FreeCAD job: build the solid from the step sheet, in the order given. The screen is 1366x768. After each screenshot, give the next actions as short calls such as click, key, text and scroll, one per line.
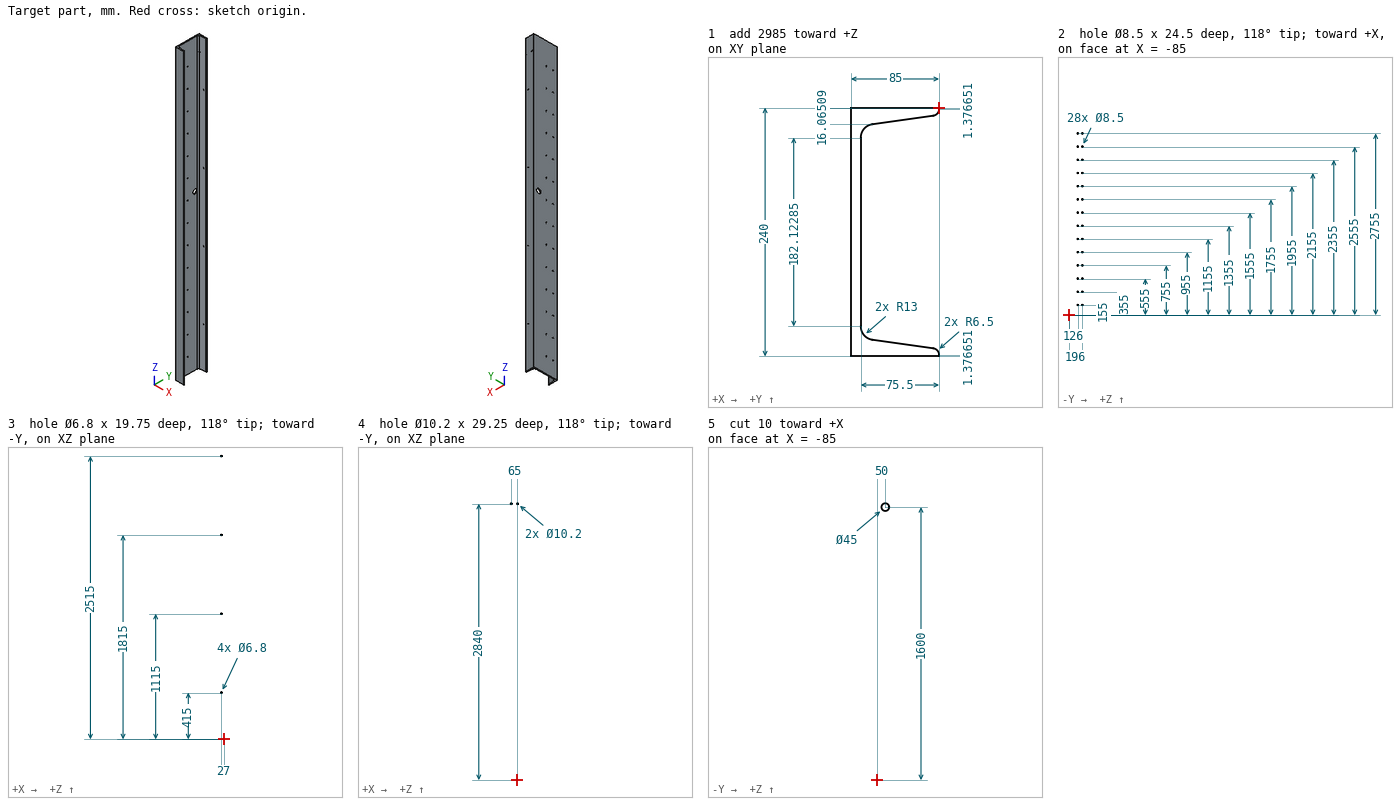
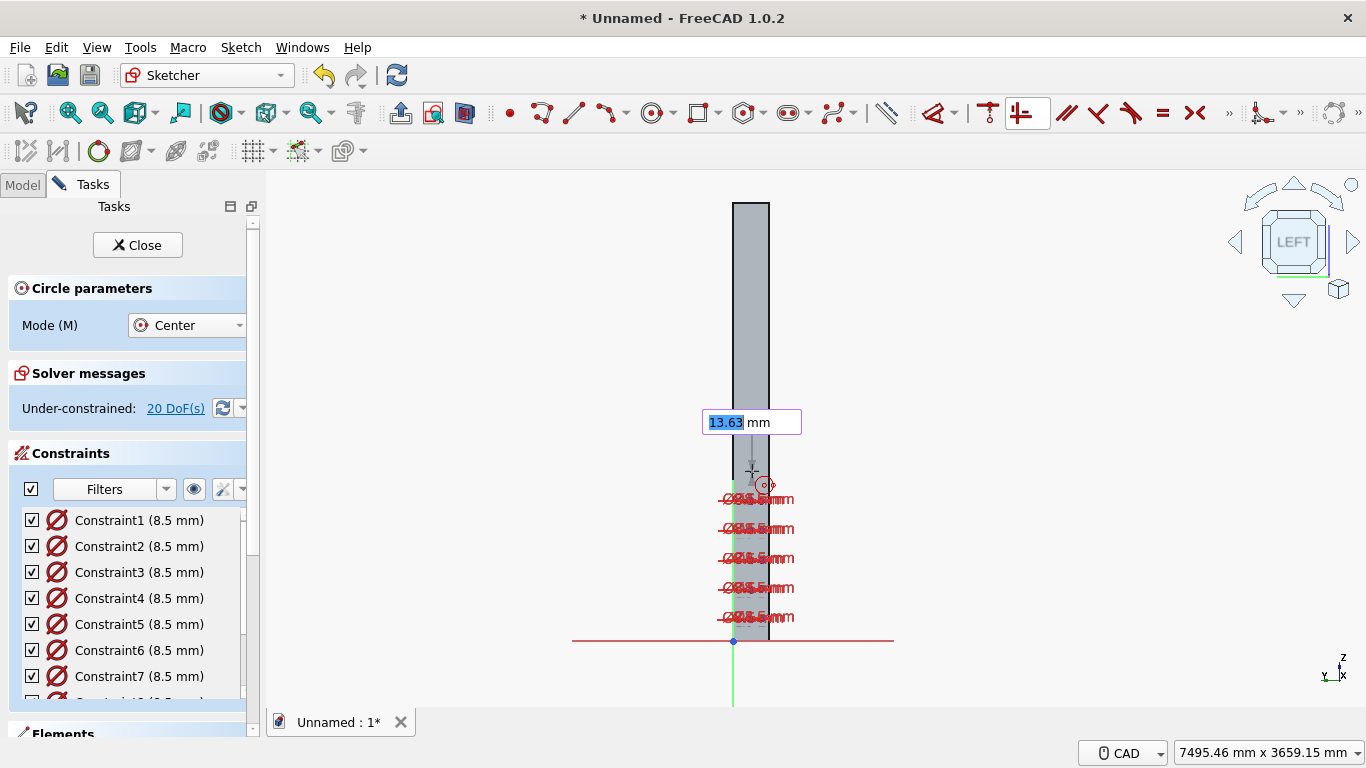
text(8.5)
key(Return)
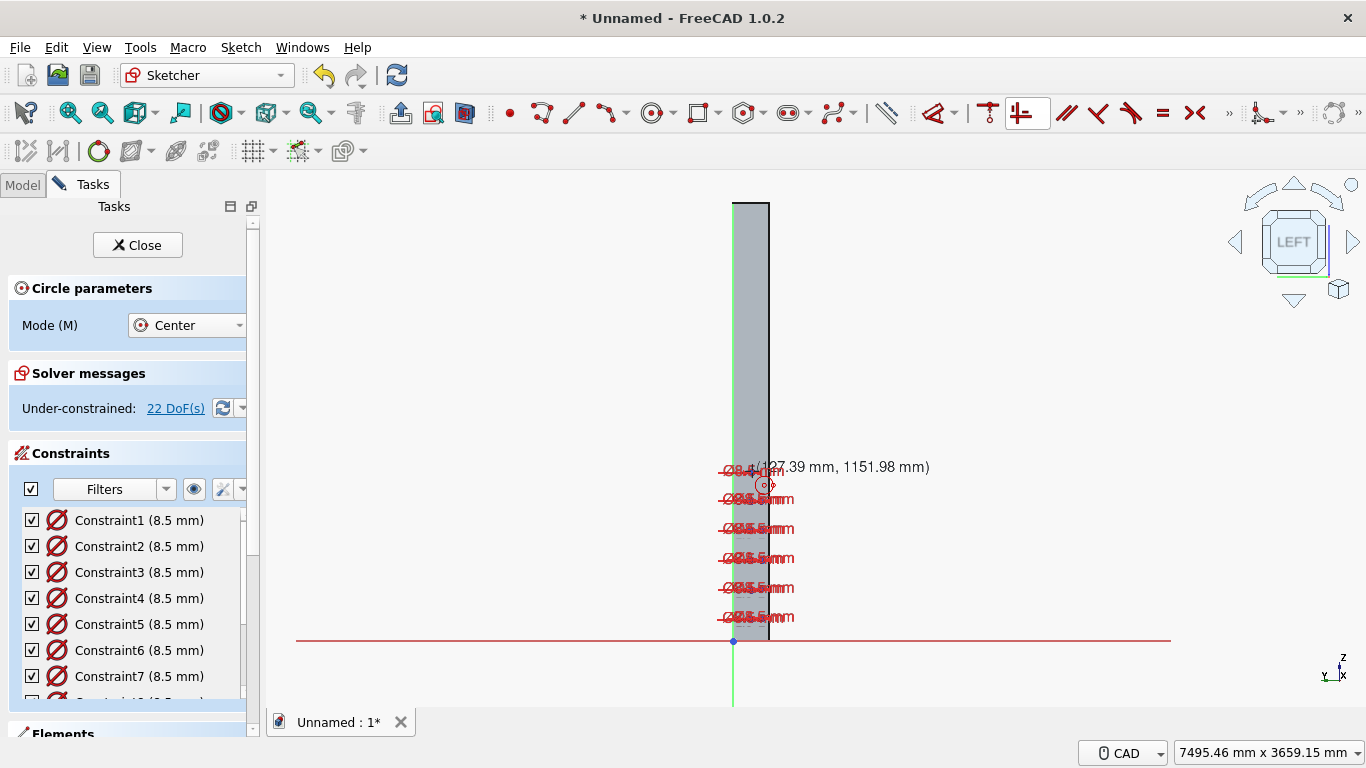
scroll(762, 472, up, 18)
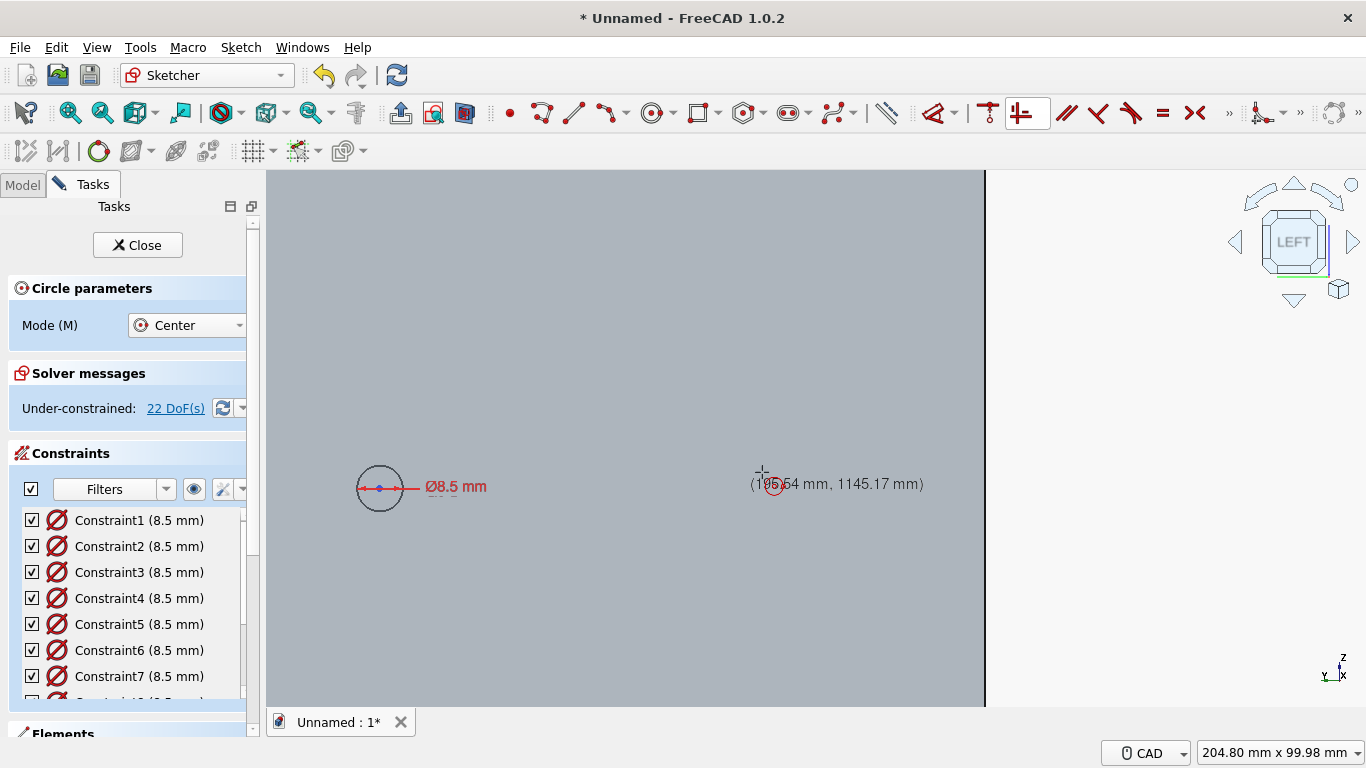
scroll(762, 472, down, 18)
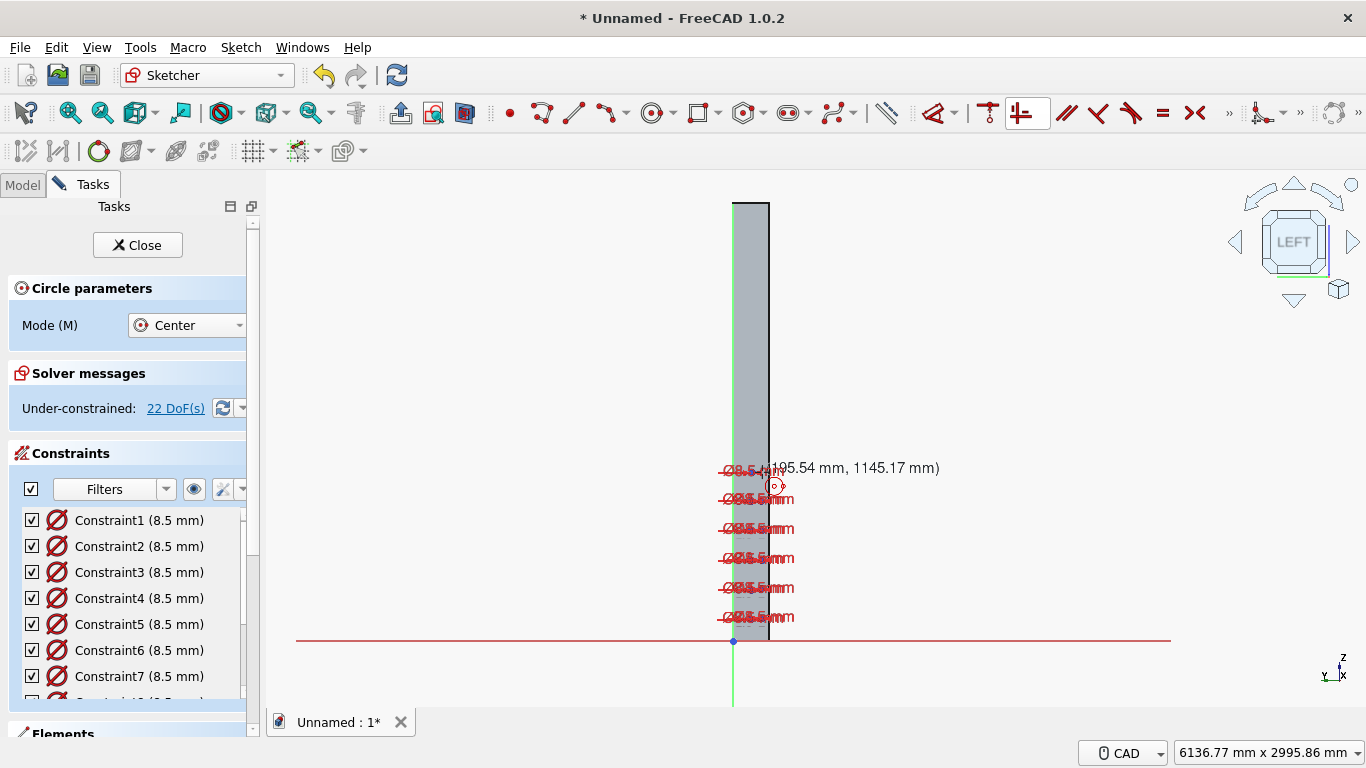
scroll(762, 472, up, 3)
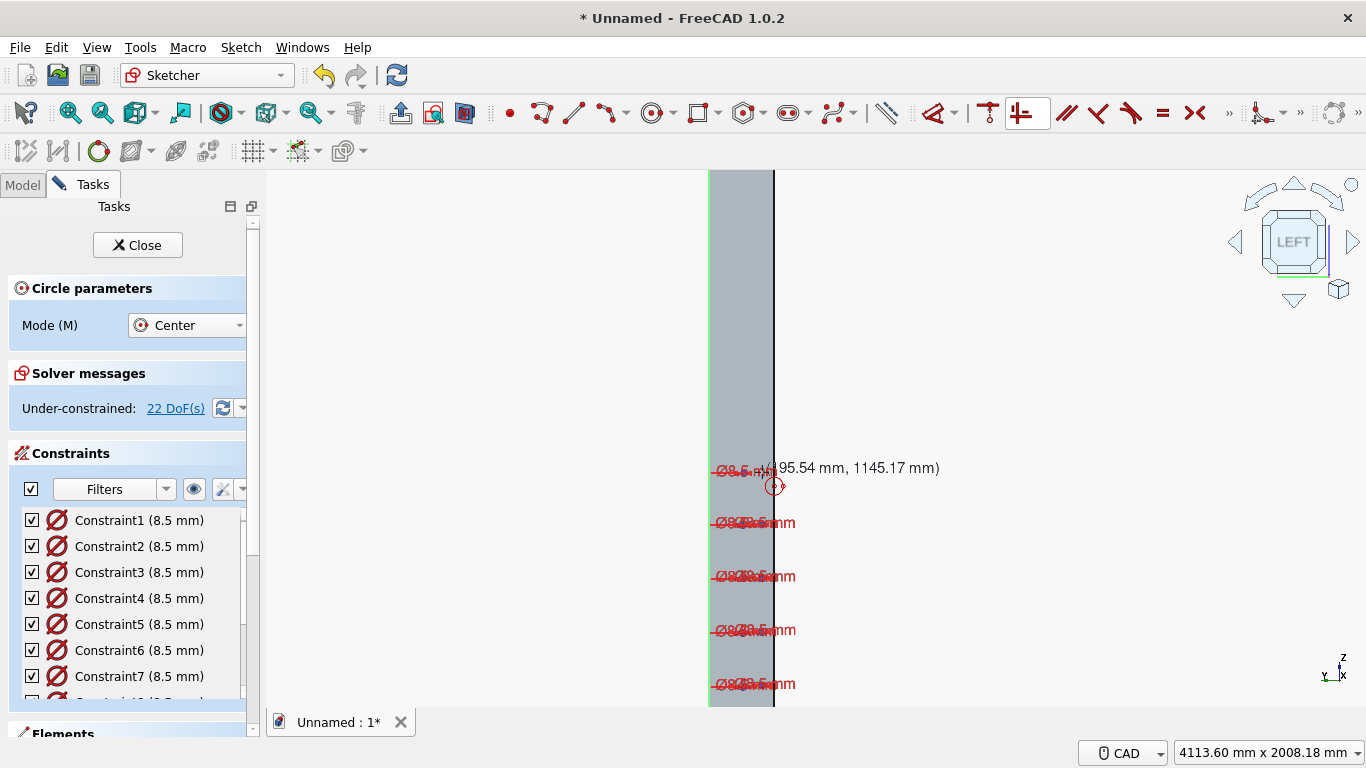
click(762, 471)
move(763, 470)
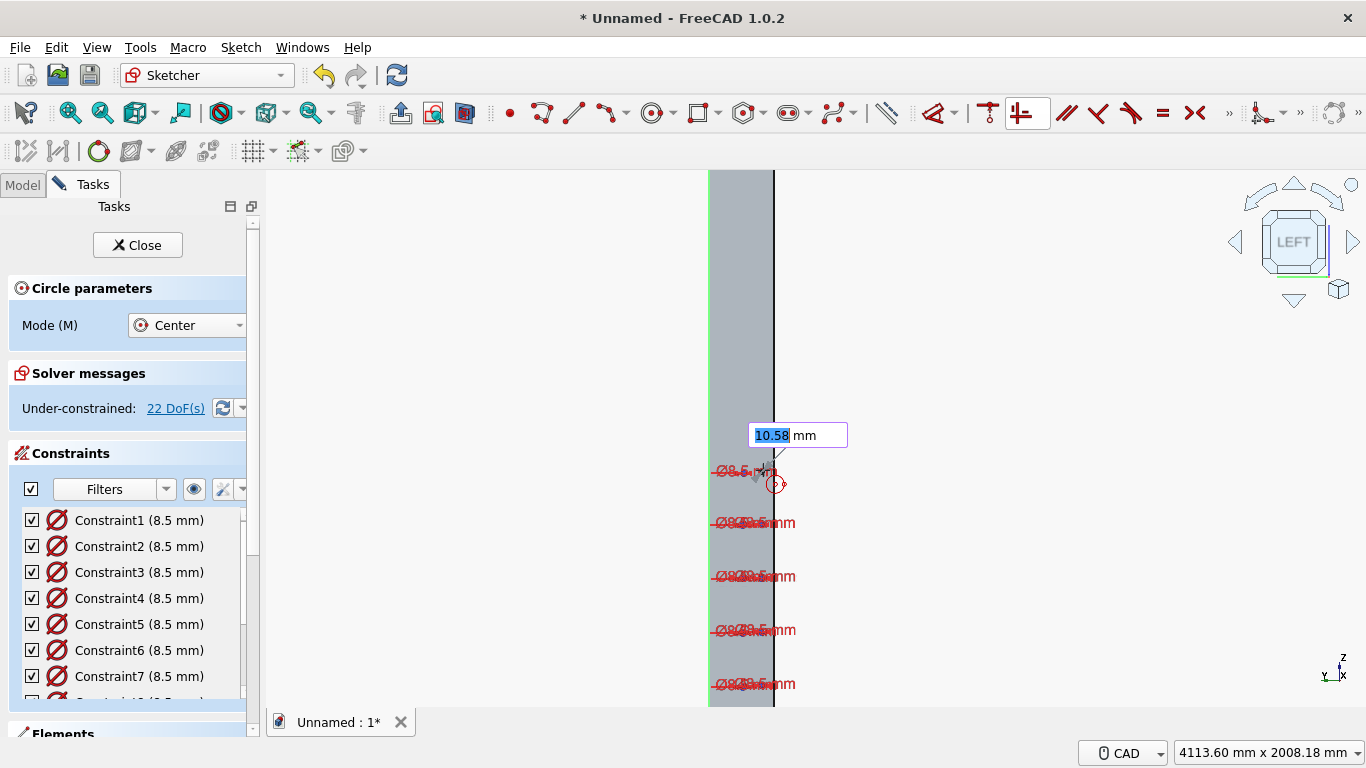
text(8.5)
key(Return)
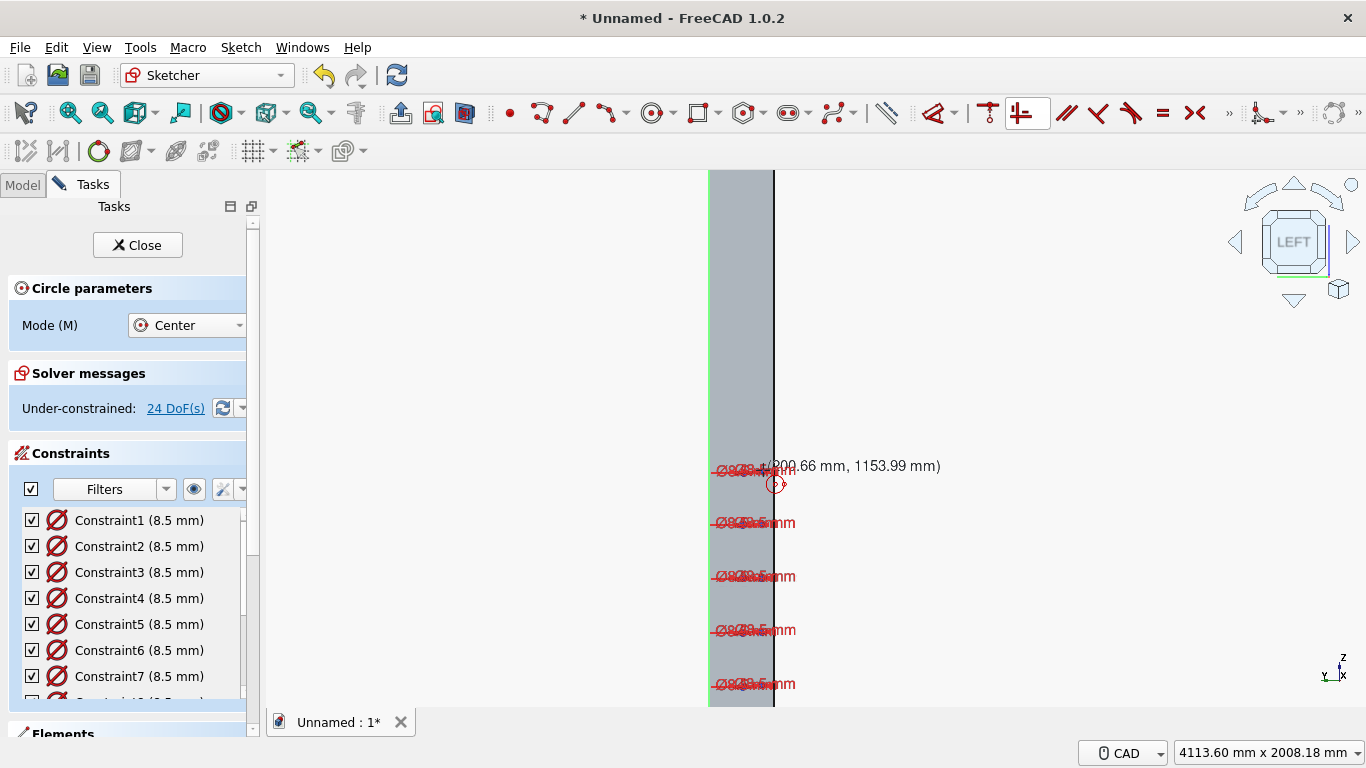
scroll(743, 417, up, 15)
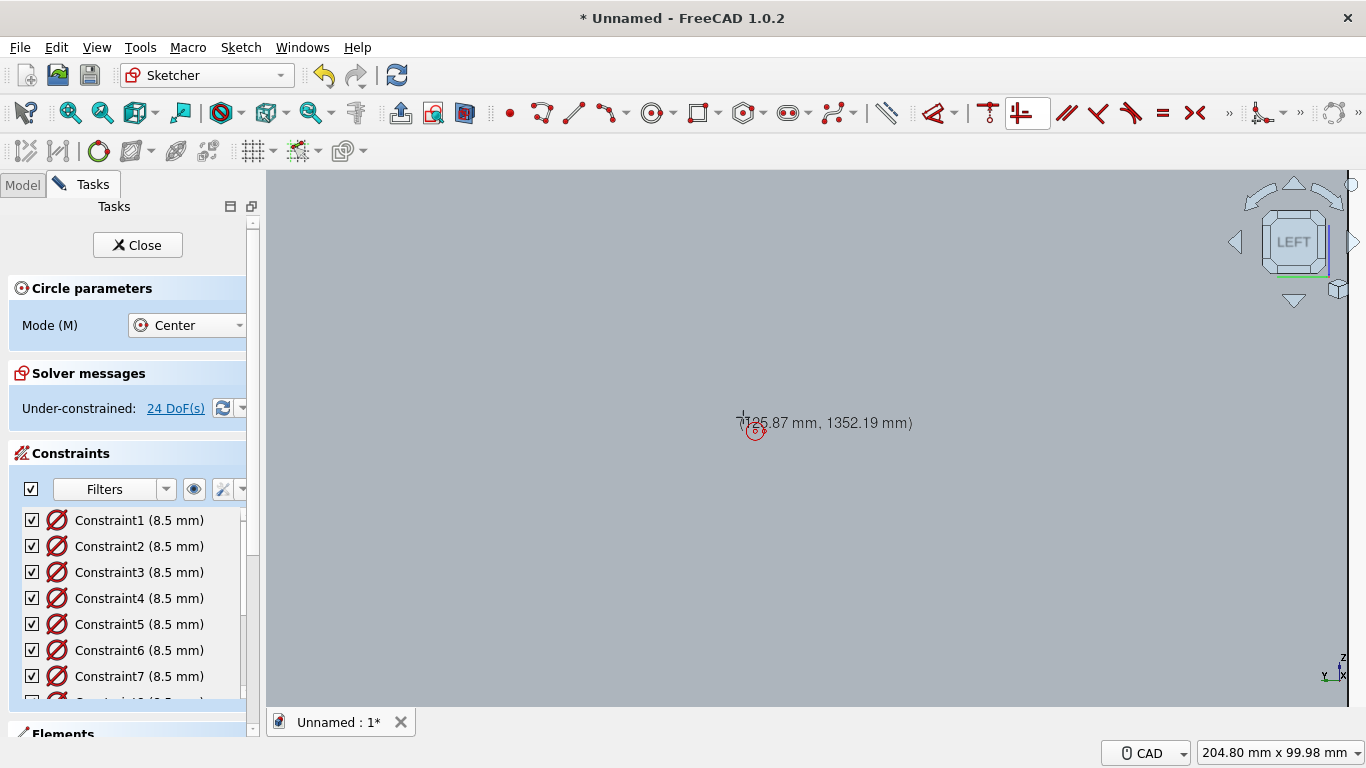
scroll(752, 443, down, 18)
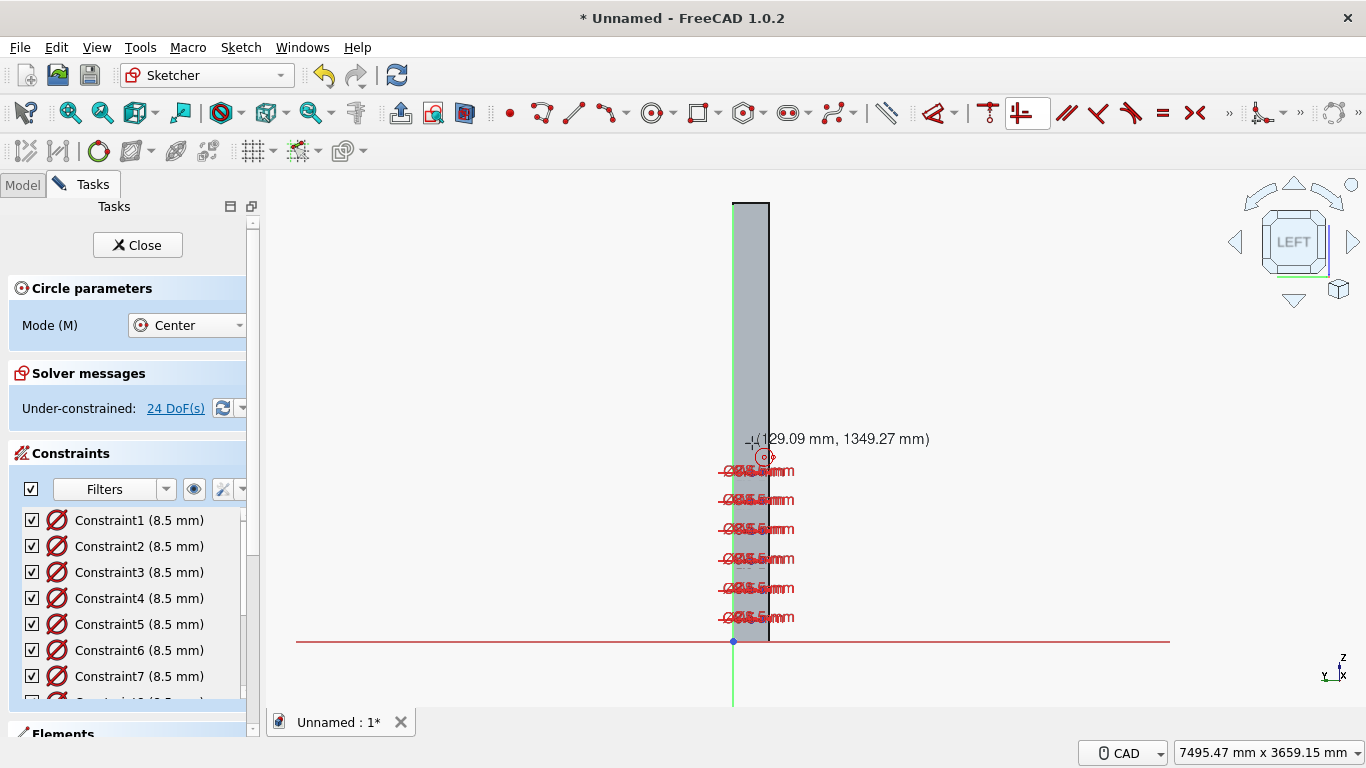
click(752, 443)
move(752, 442)